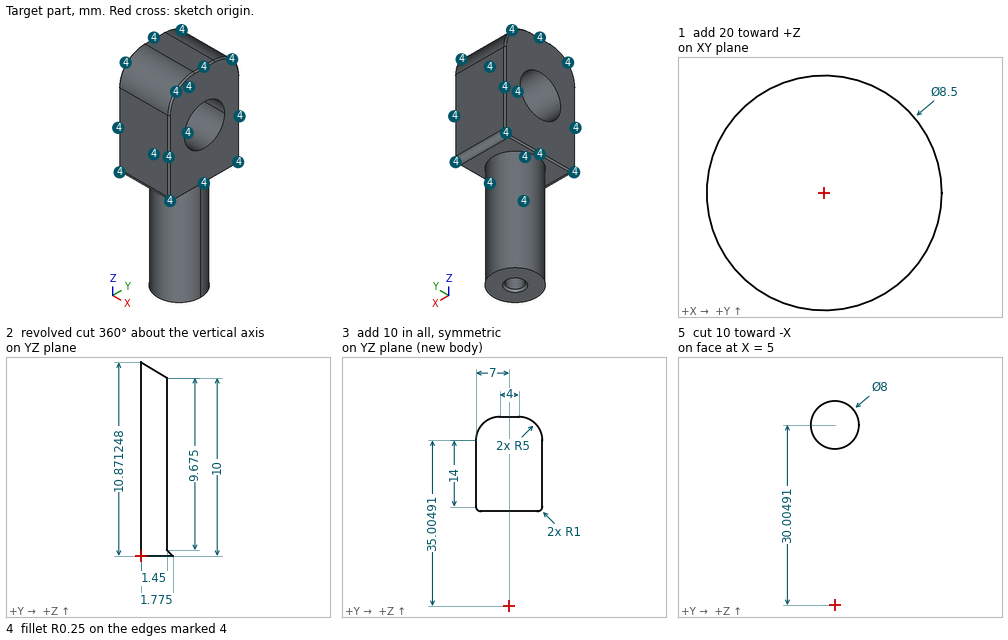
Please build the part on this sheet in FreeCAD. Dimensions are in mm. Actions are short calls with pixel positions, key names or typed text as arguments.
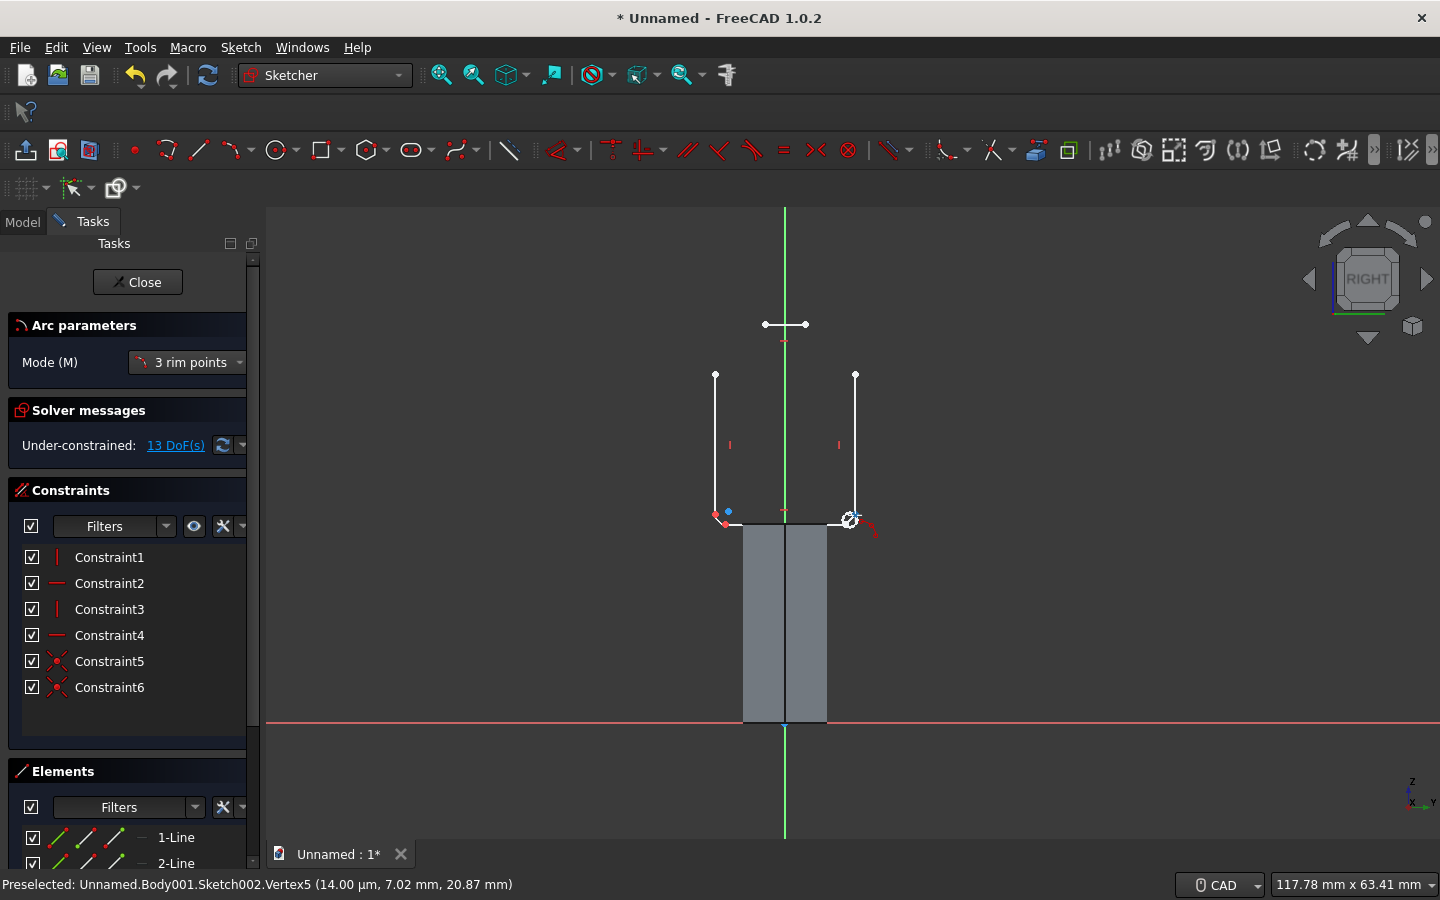
scroll(852, 521, up, 9)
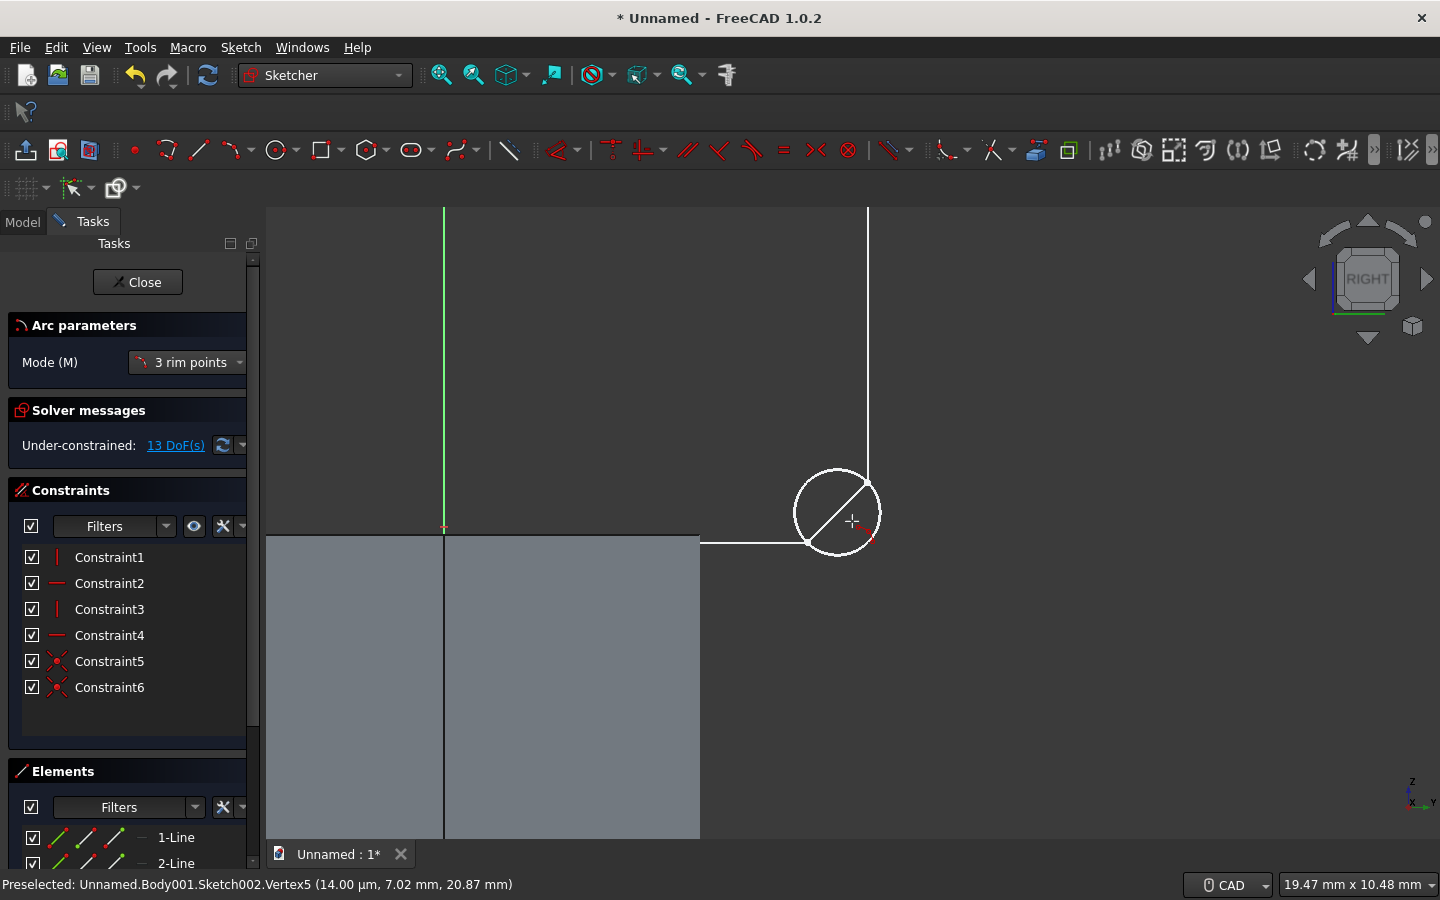
click(849, 517)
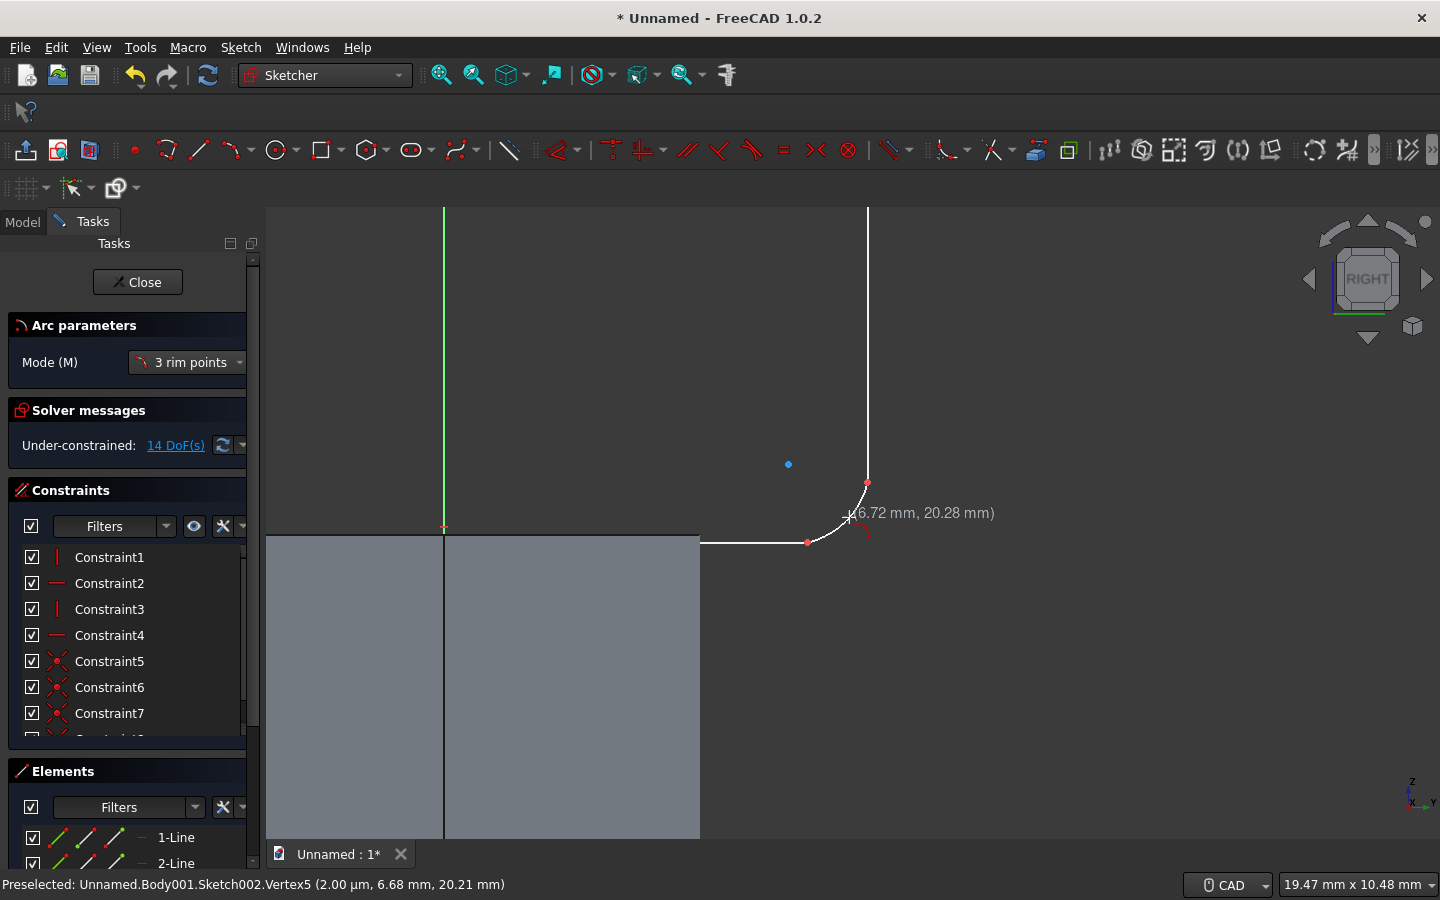
scroll(852, 521, down, 9)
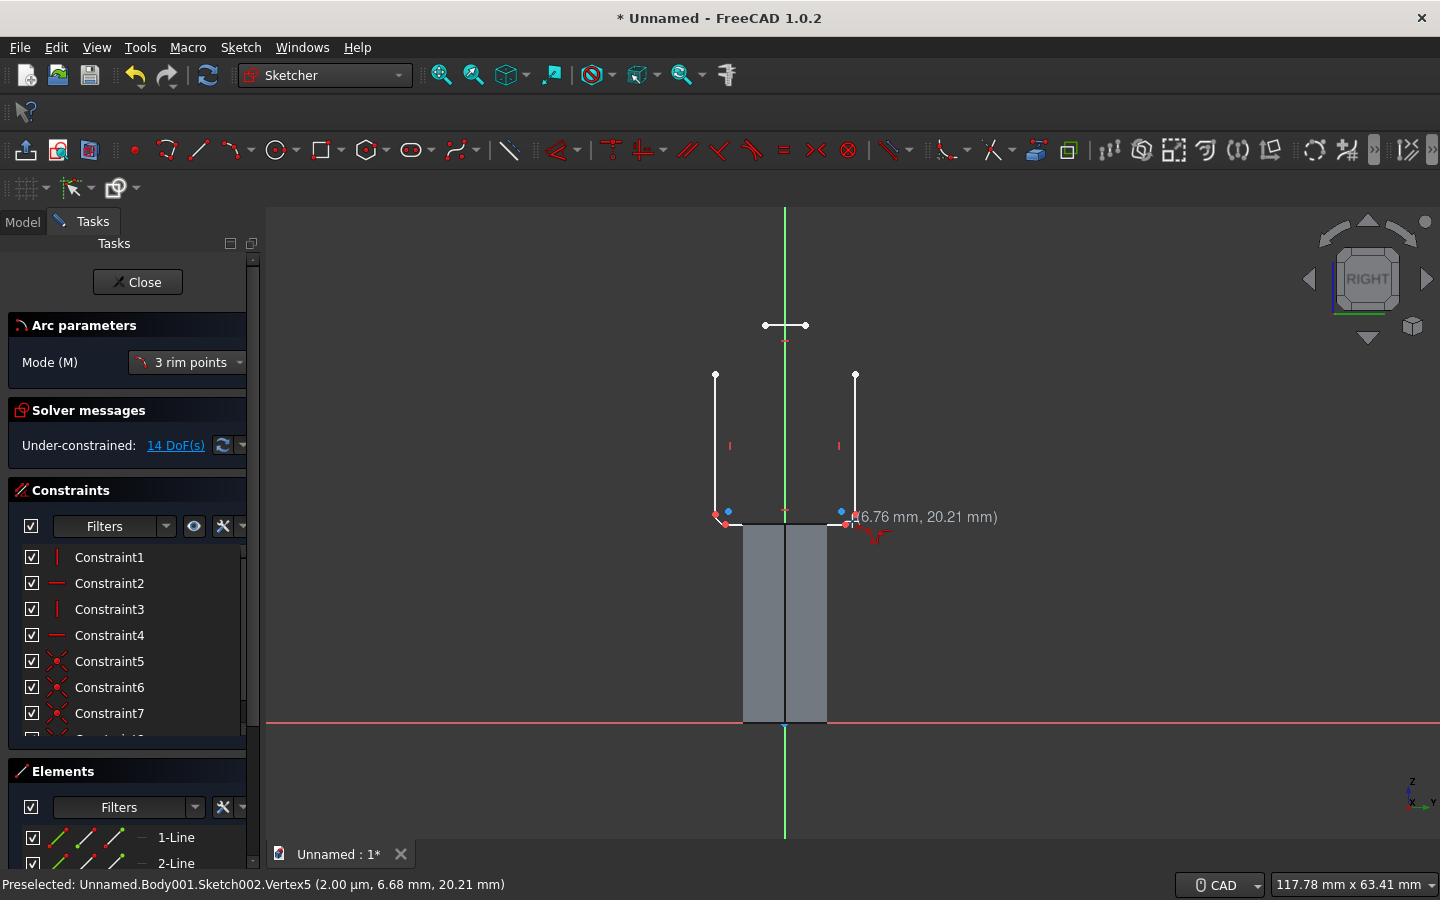
click(855, 375)
click(805, 325)
click(840, 339)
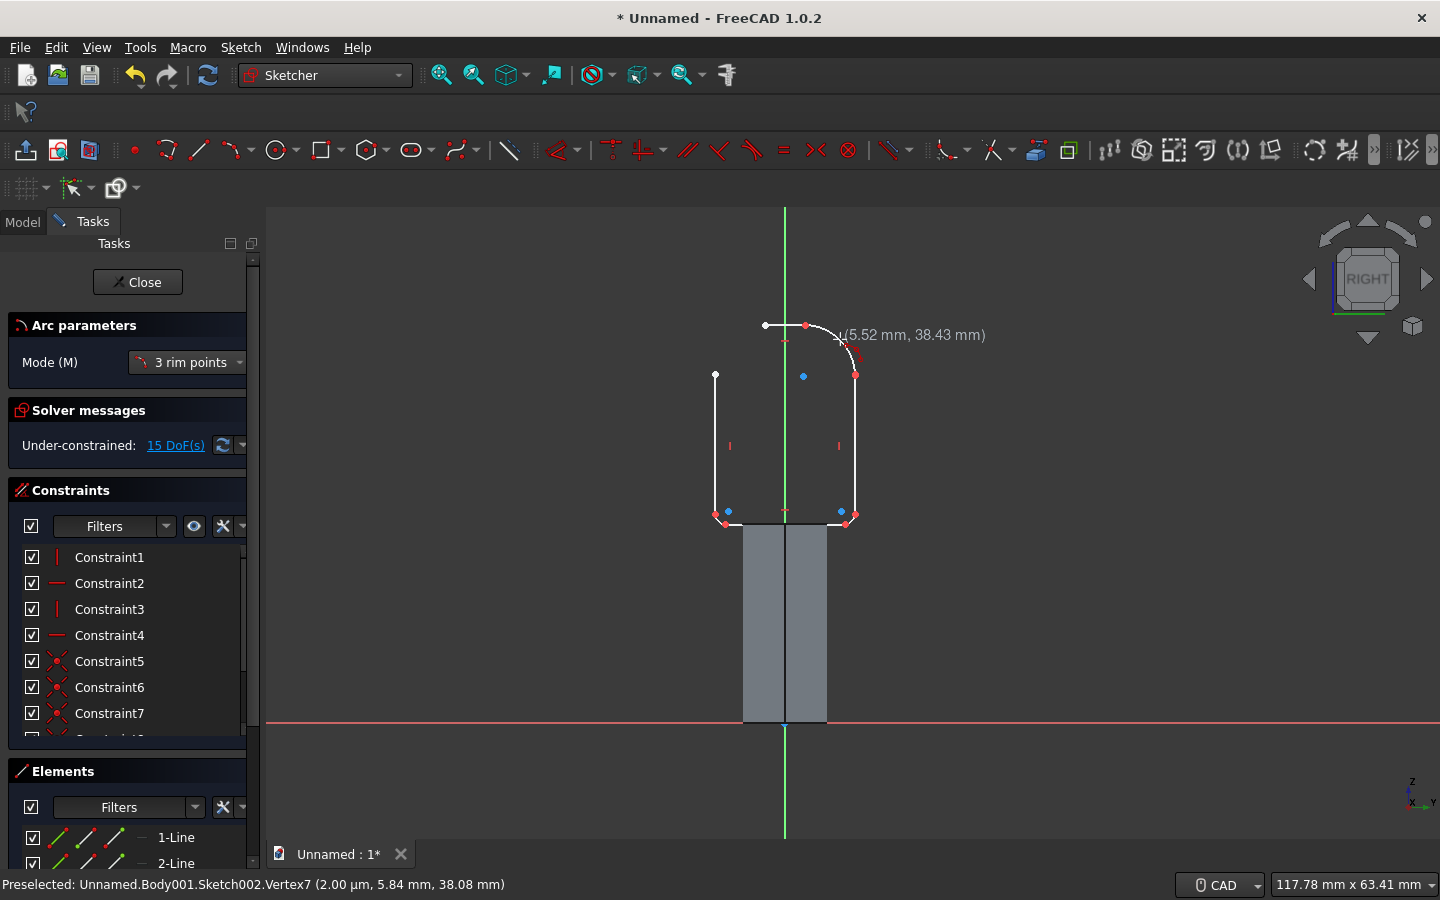
click(765, 325)
click(715, 375)
click(730, 339)
key(Escape)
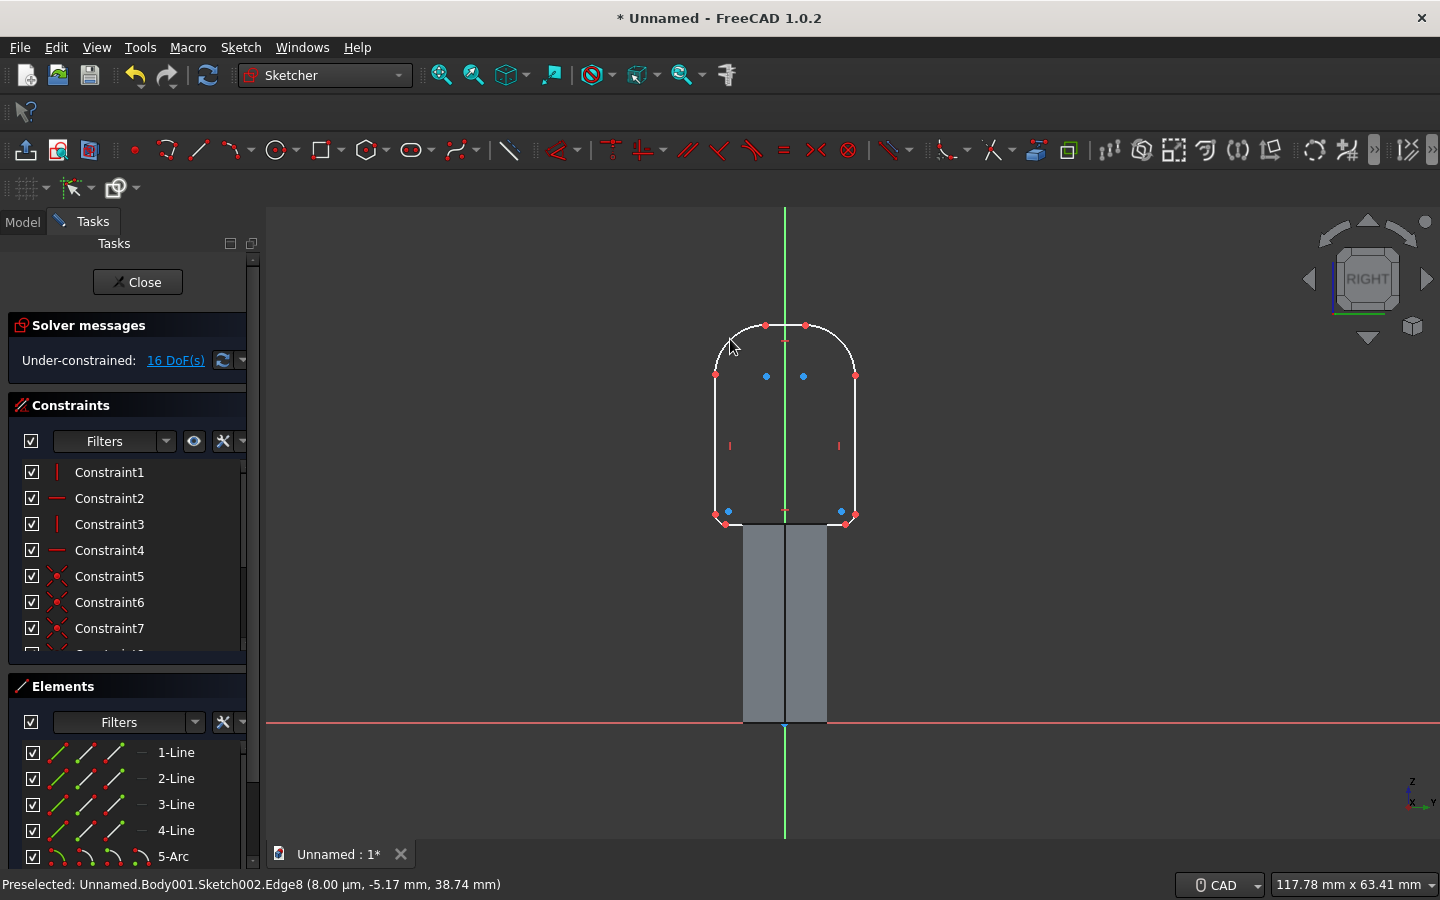
click(715, 417)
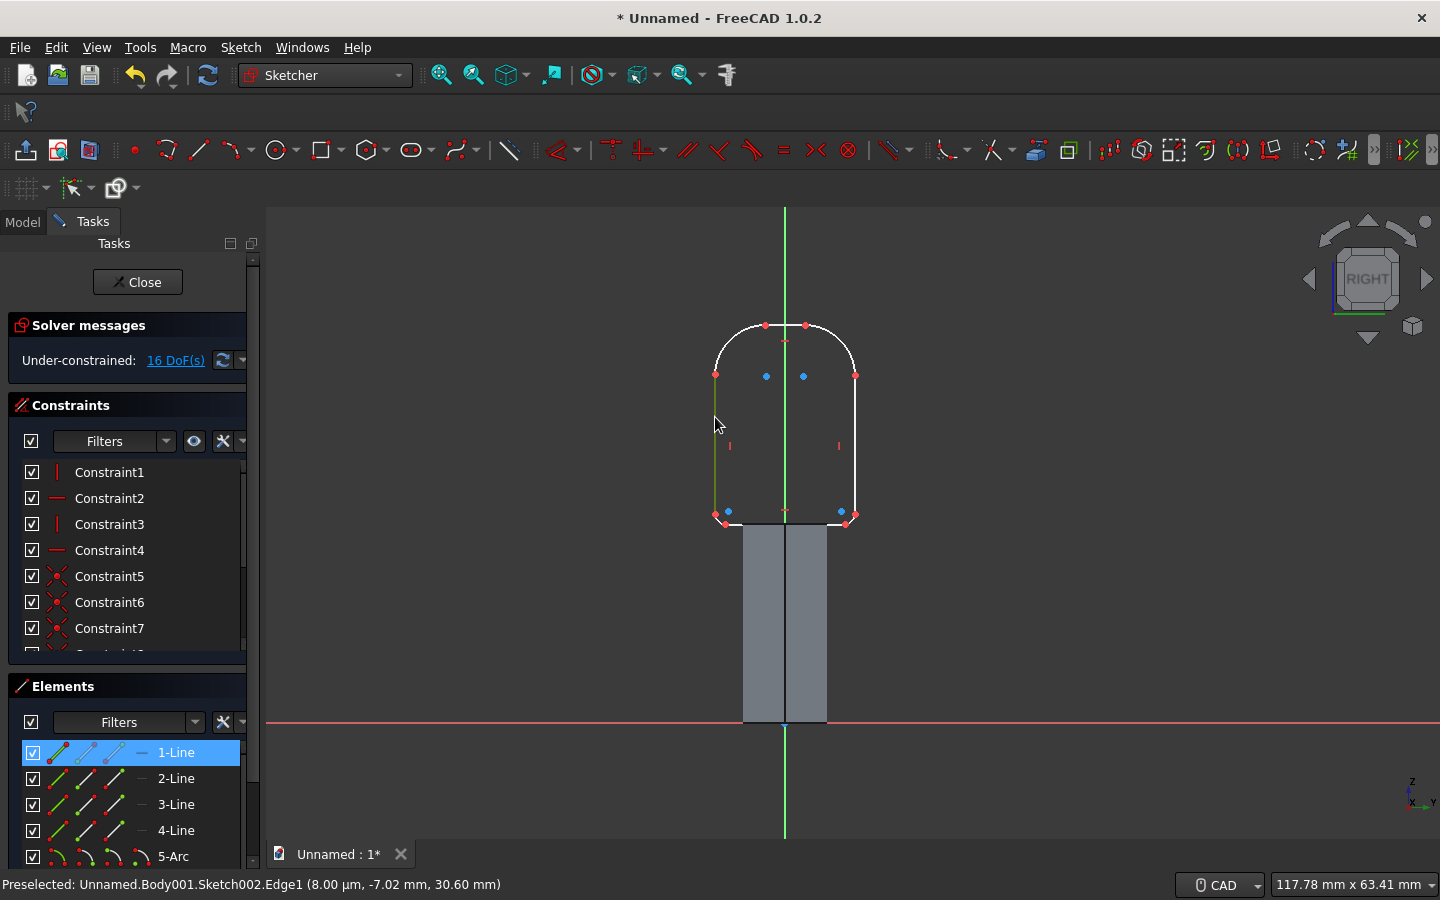
scroll(719, 521, up, 4)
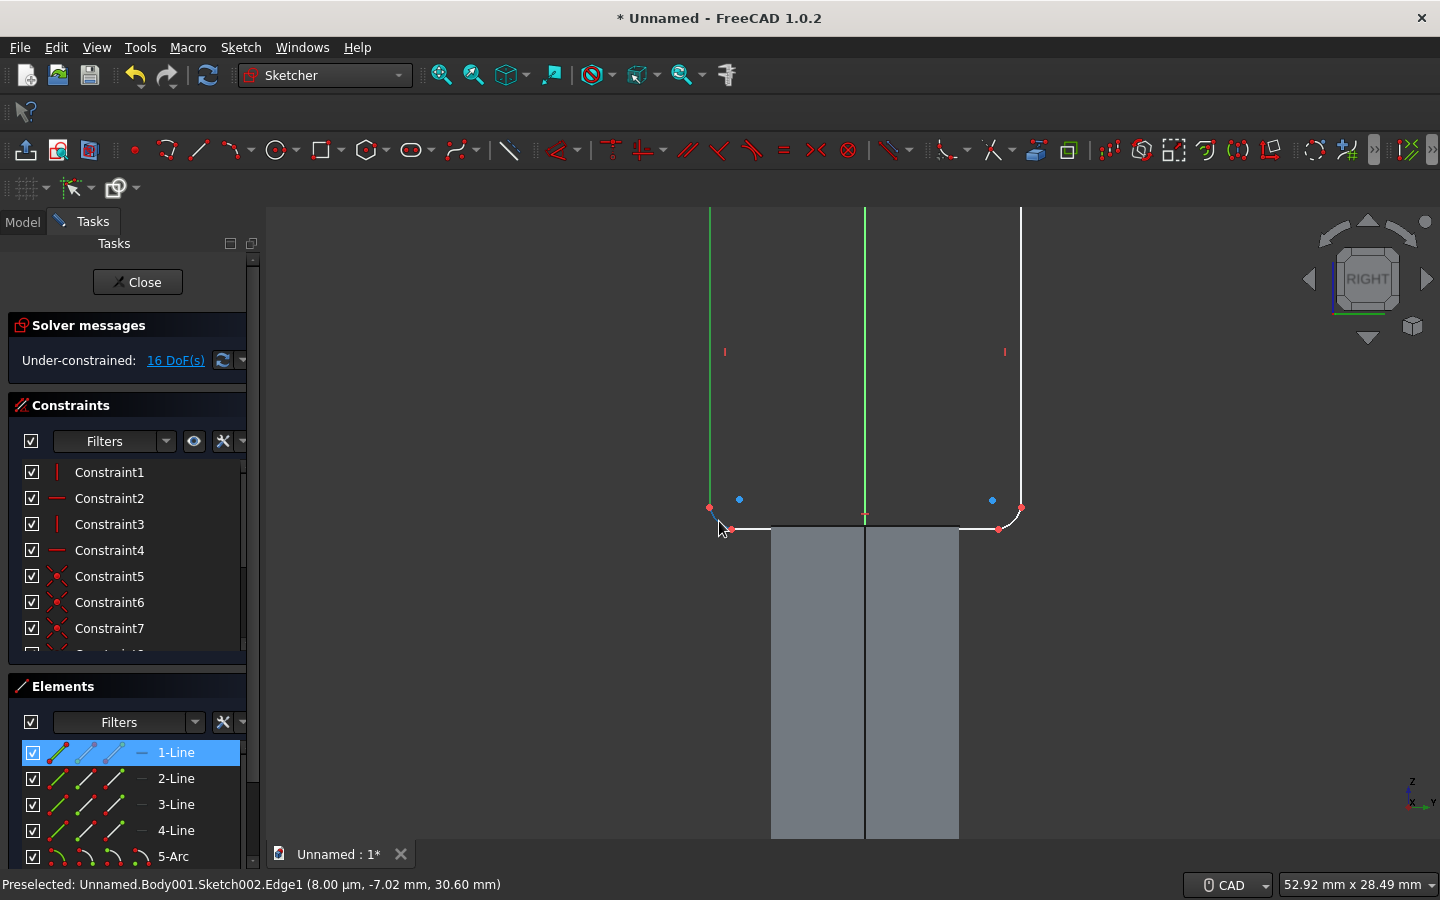
click(718, 521)